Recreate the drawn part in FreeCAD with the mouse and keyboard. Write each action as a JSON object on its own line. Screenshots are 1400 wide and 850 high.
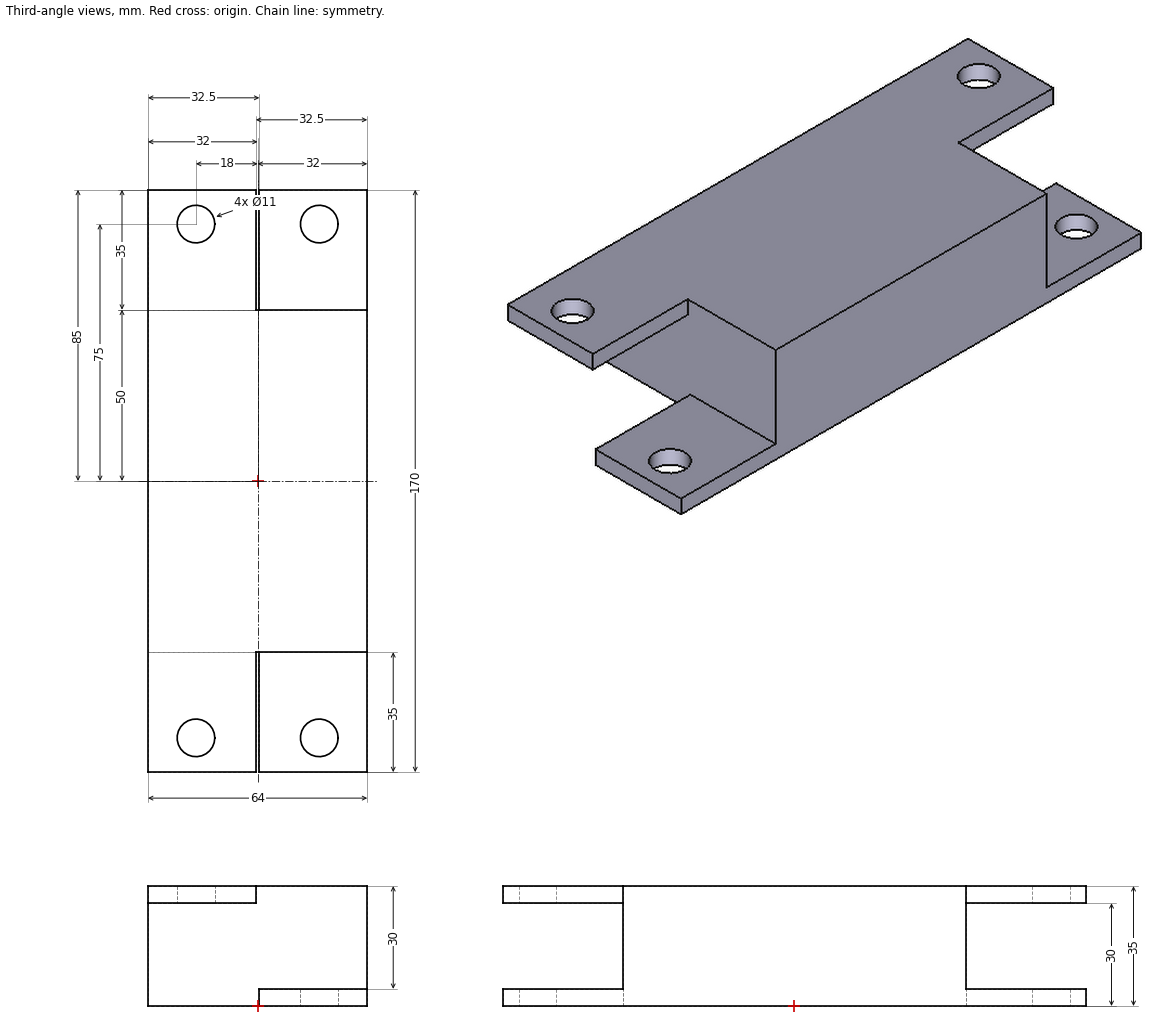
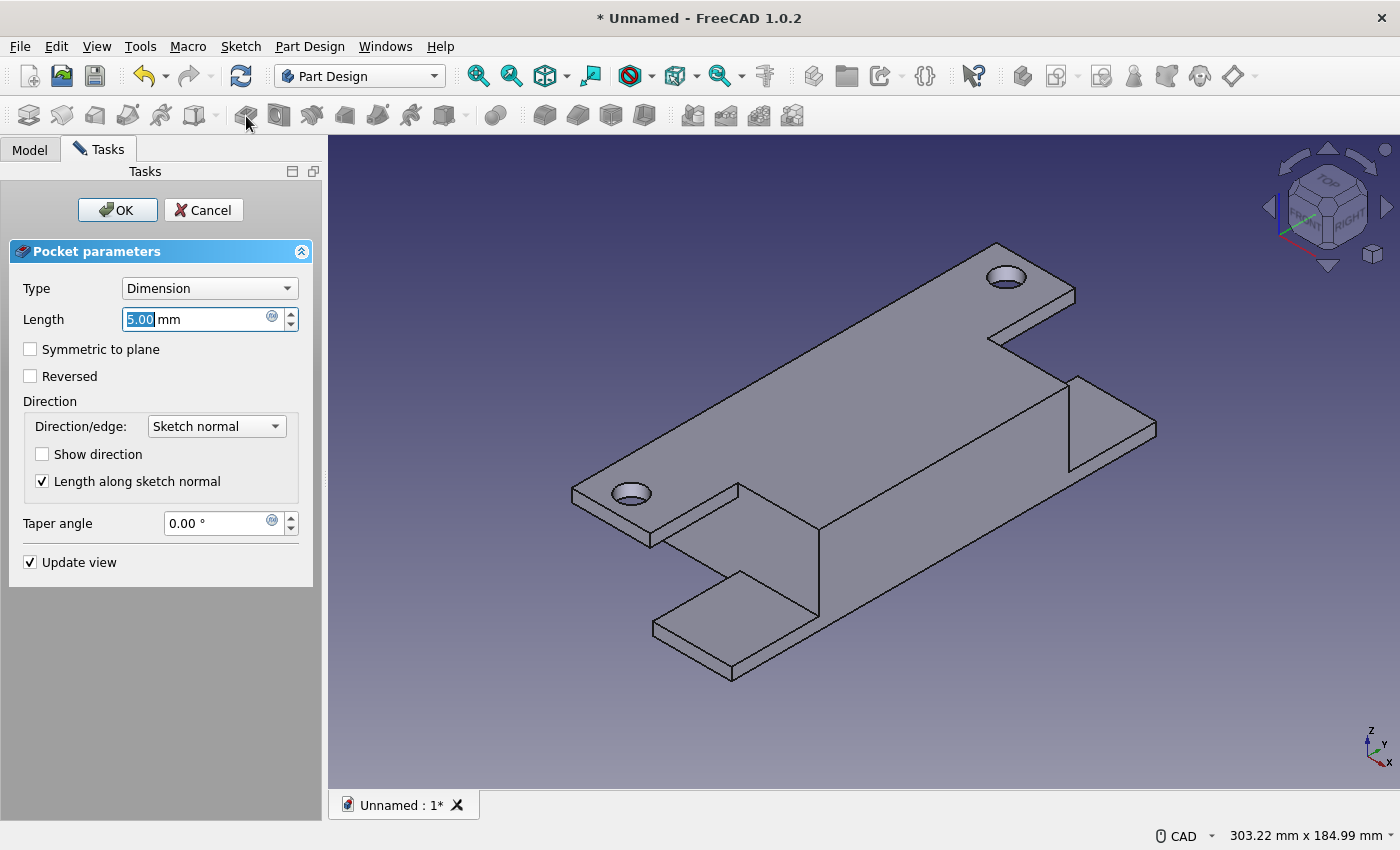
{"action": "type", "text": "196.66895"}
{"action": "key", "text": "Tab"}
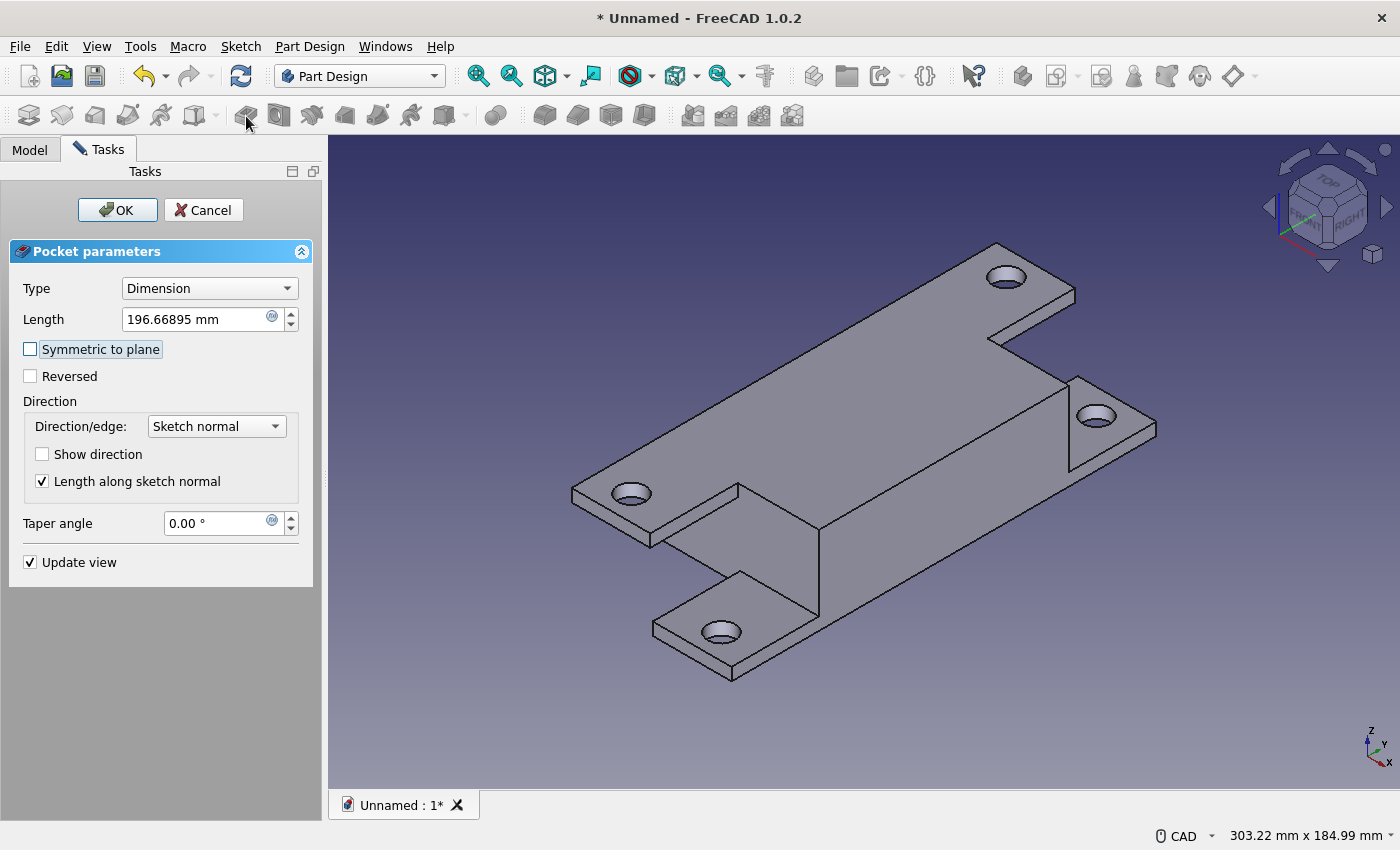
{"action": "left_click", "coordinate": [31, 349]}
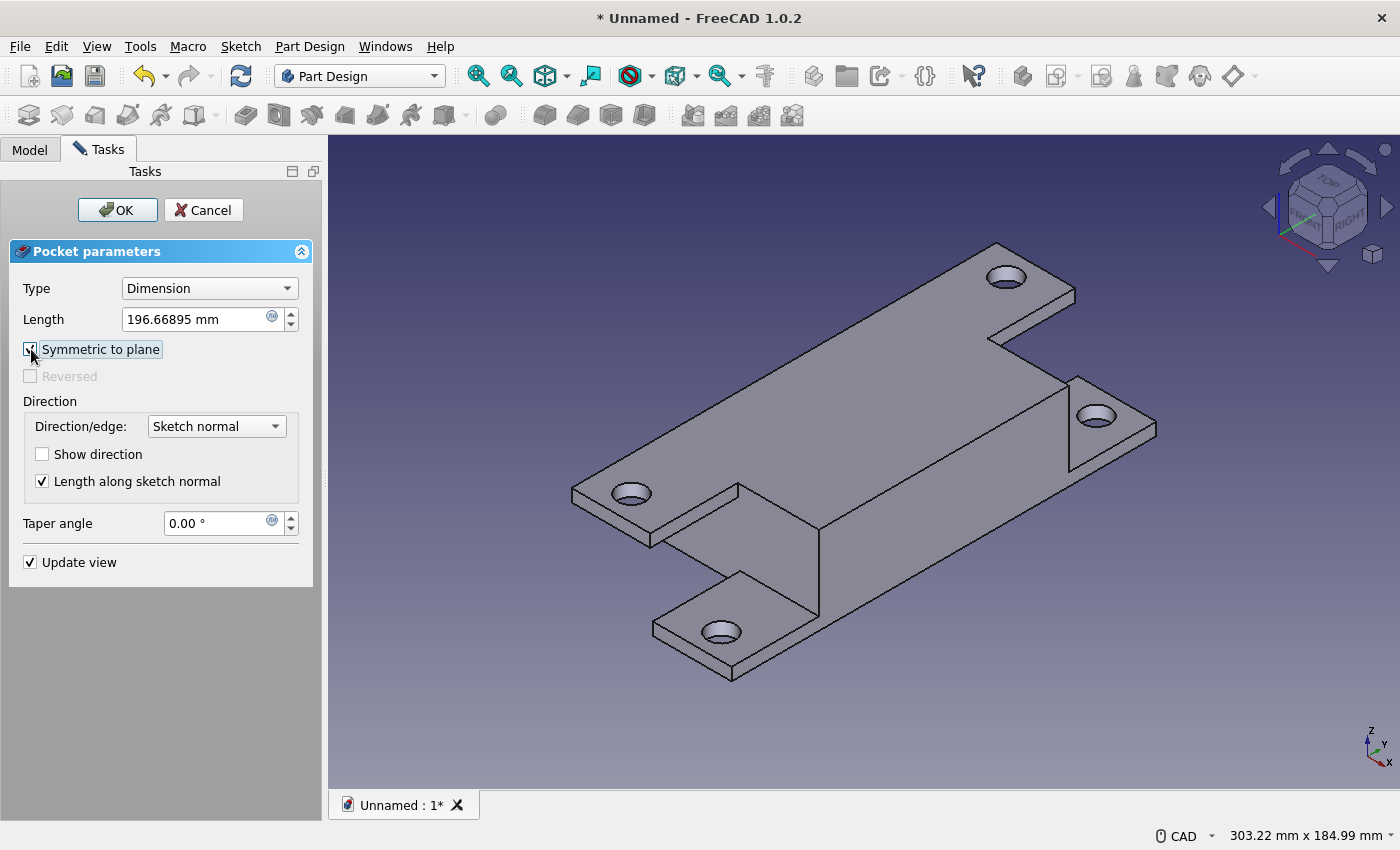
{"action": "left_click", "coordinate": [118, 210]}